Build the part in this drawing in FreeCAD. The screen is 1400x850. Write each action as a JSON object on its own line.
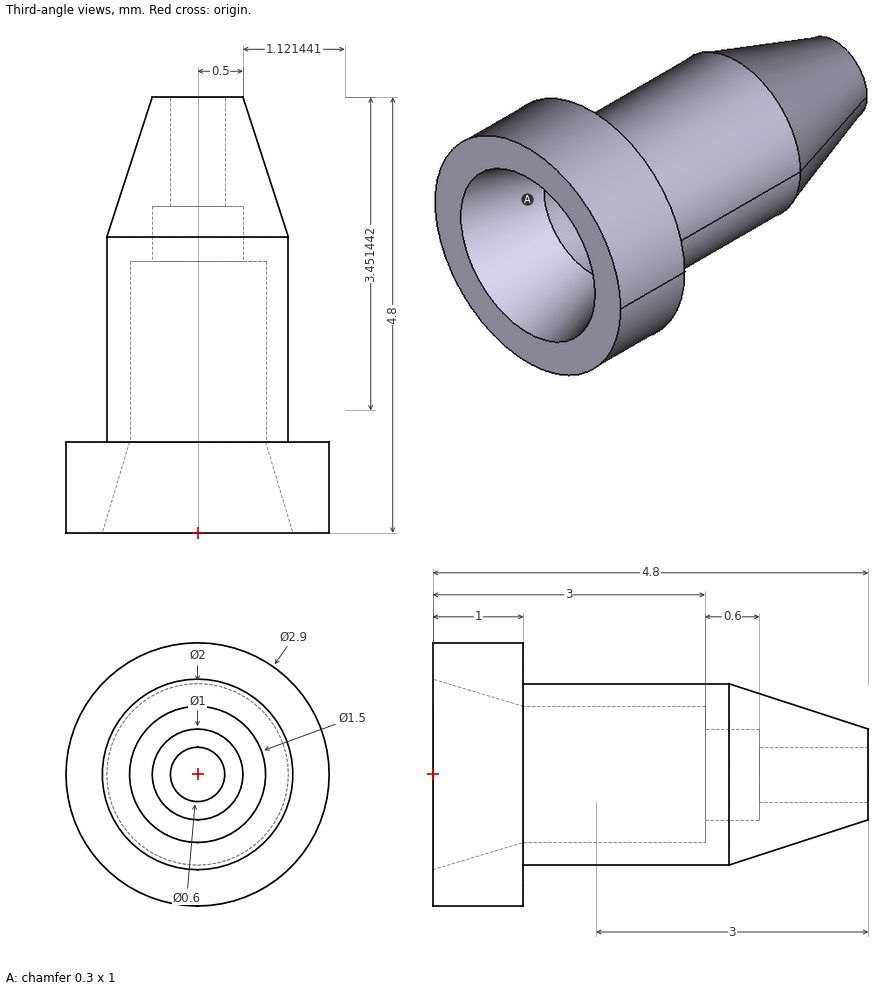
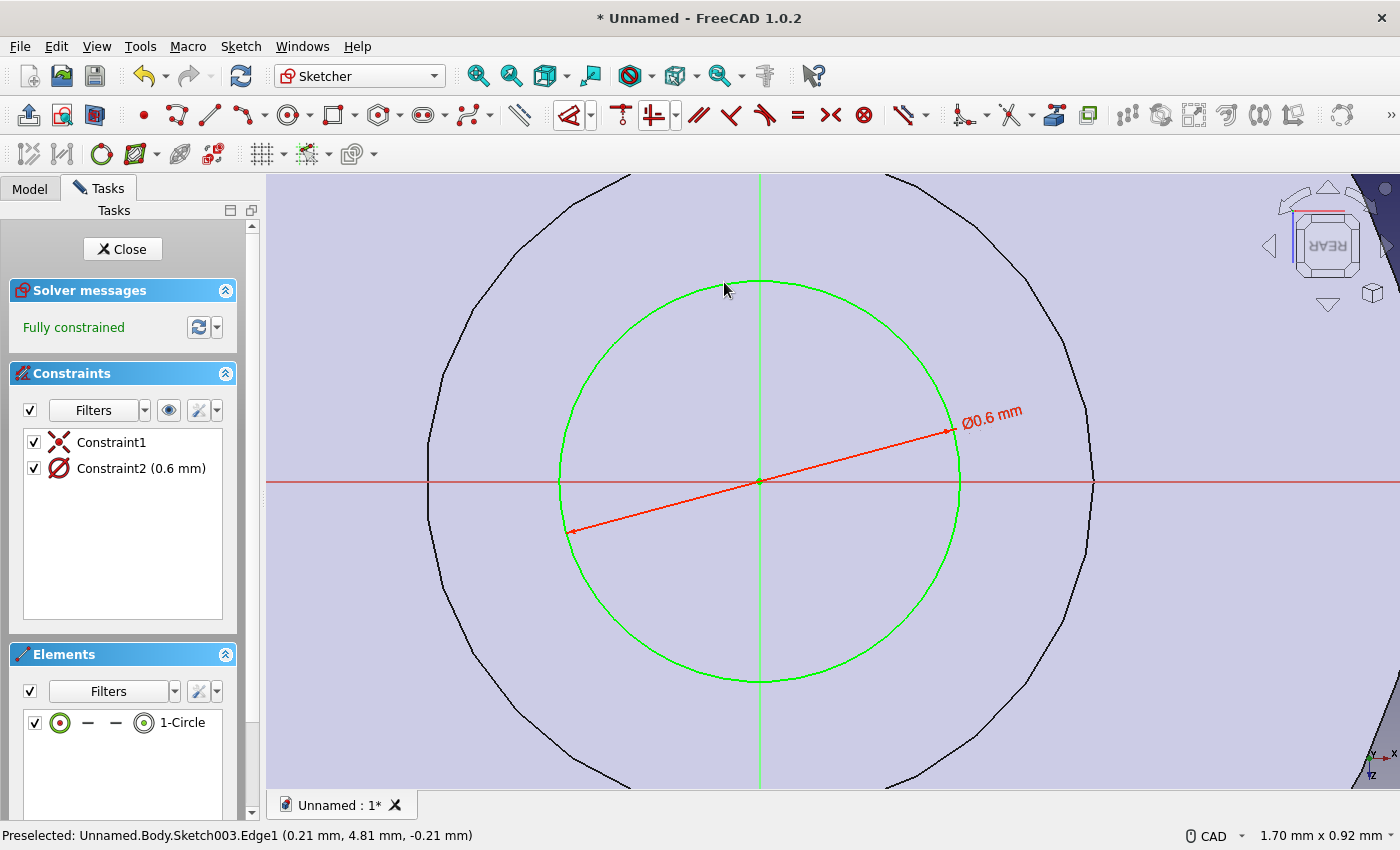
{"action": "left_click", "coordinate": [123, 249]}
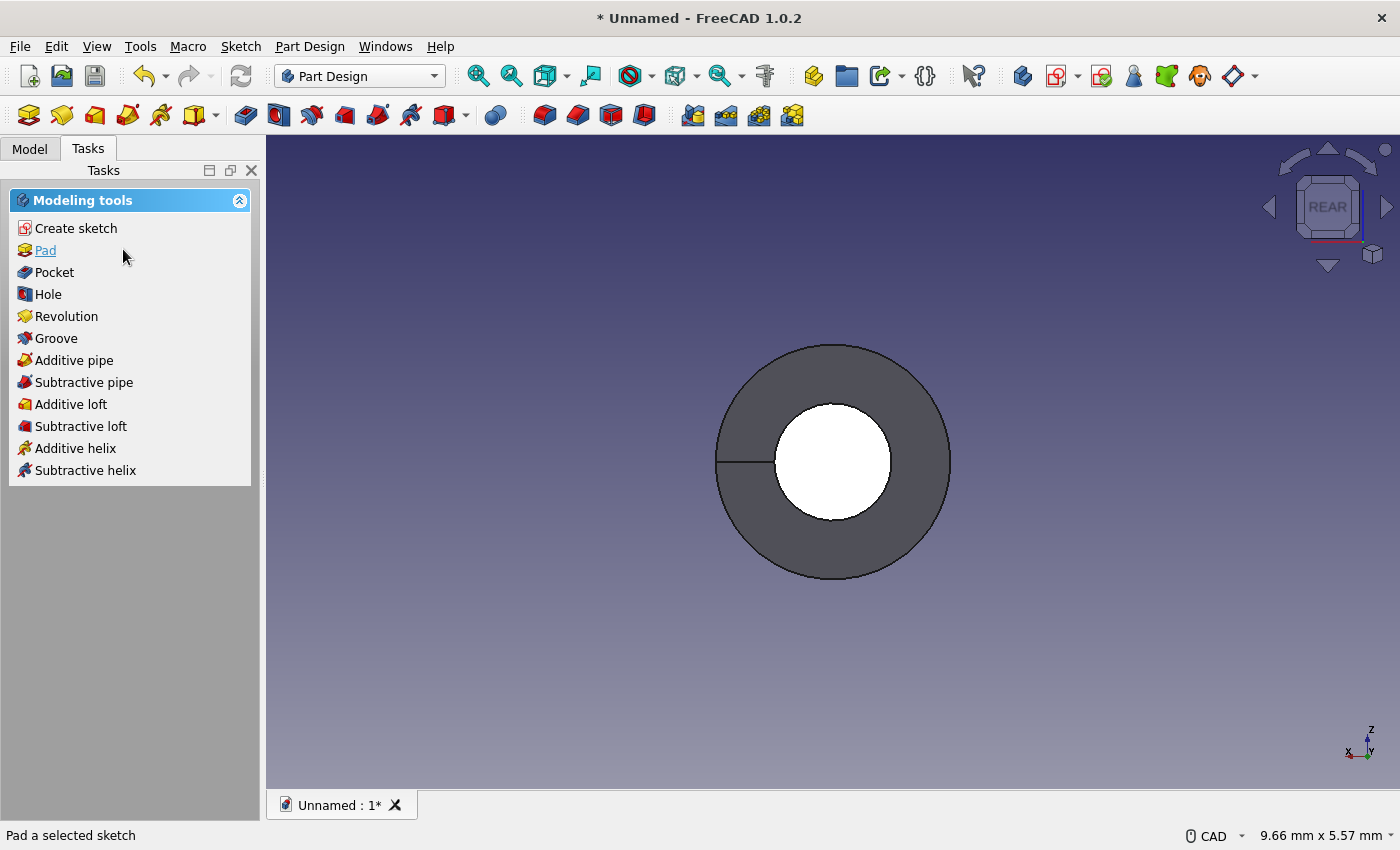
{"action": "left_click", "coordinate": [246, 116]}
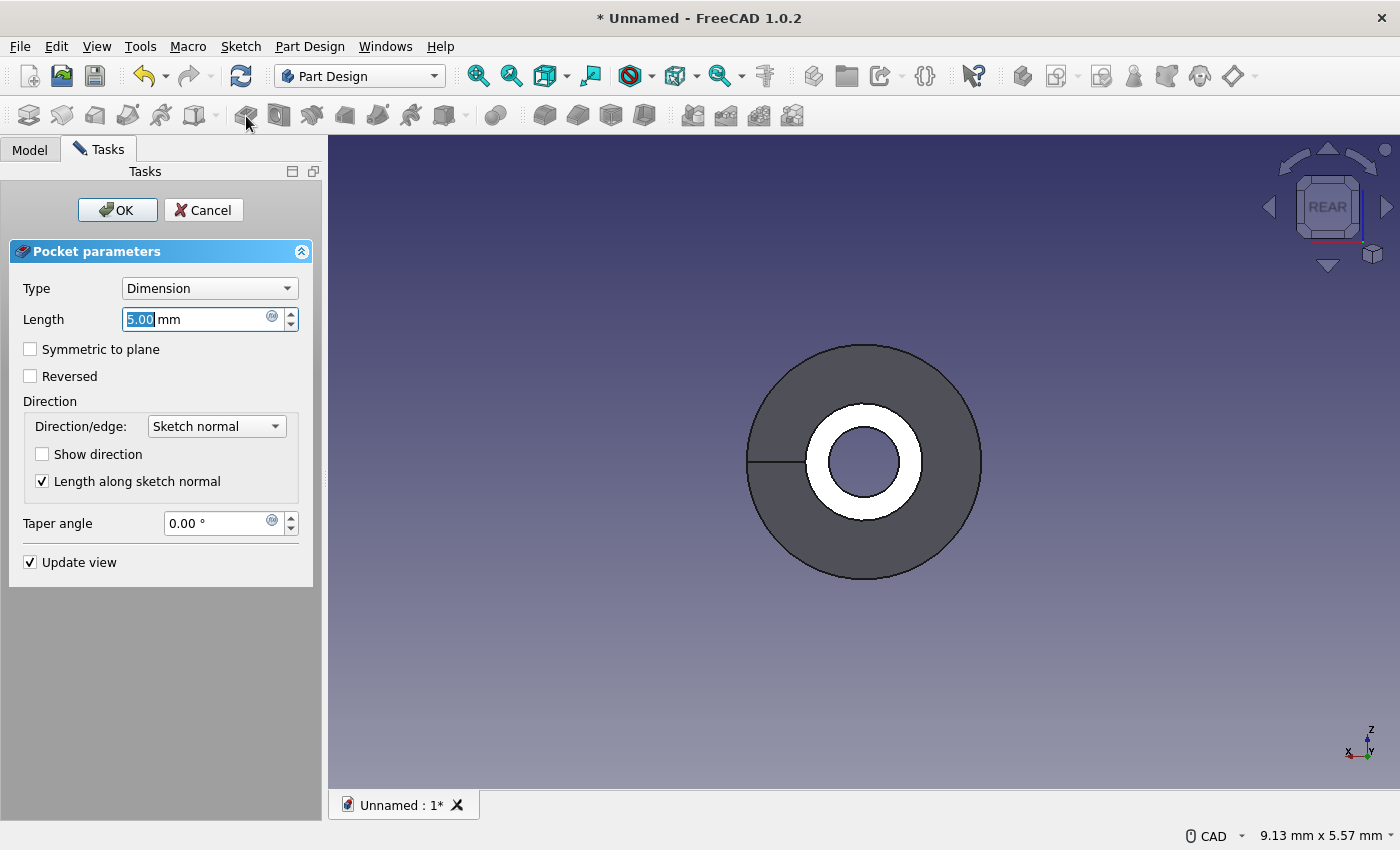
{"action": "type", "text": "3"}
{"action": "key", "text": "Tab"}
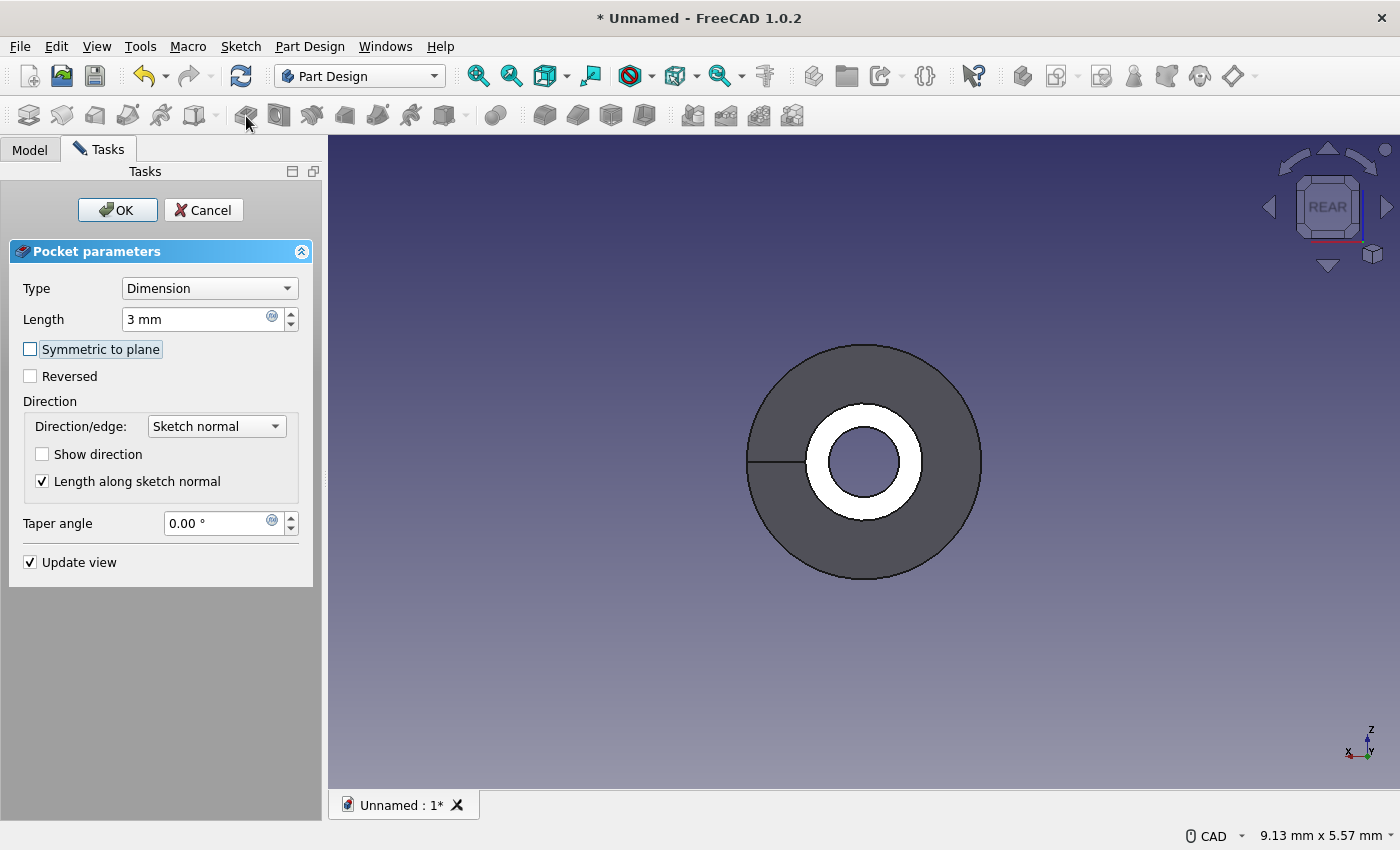
{"action": "left_click", "coordinate": [118, 210]}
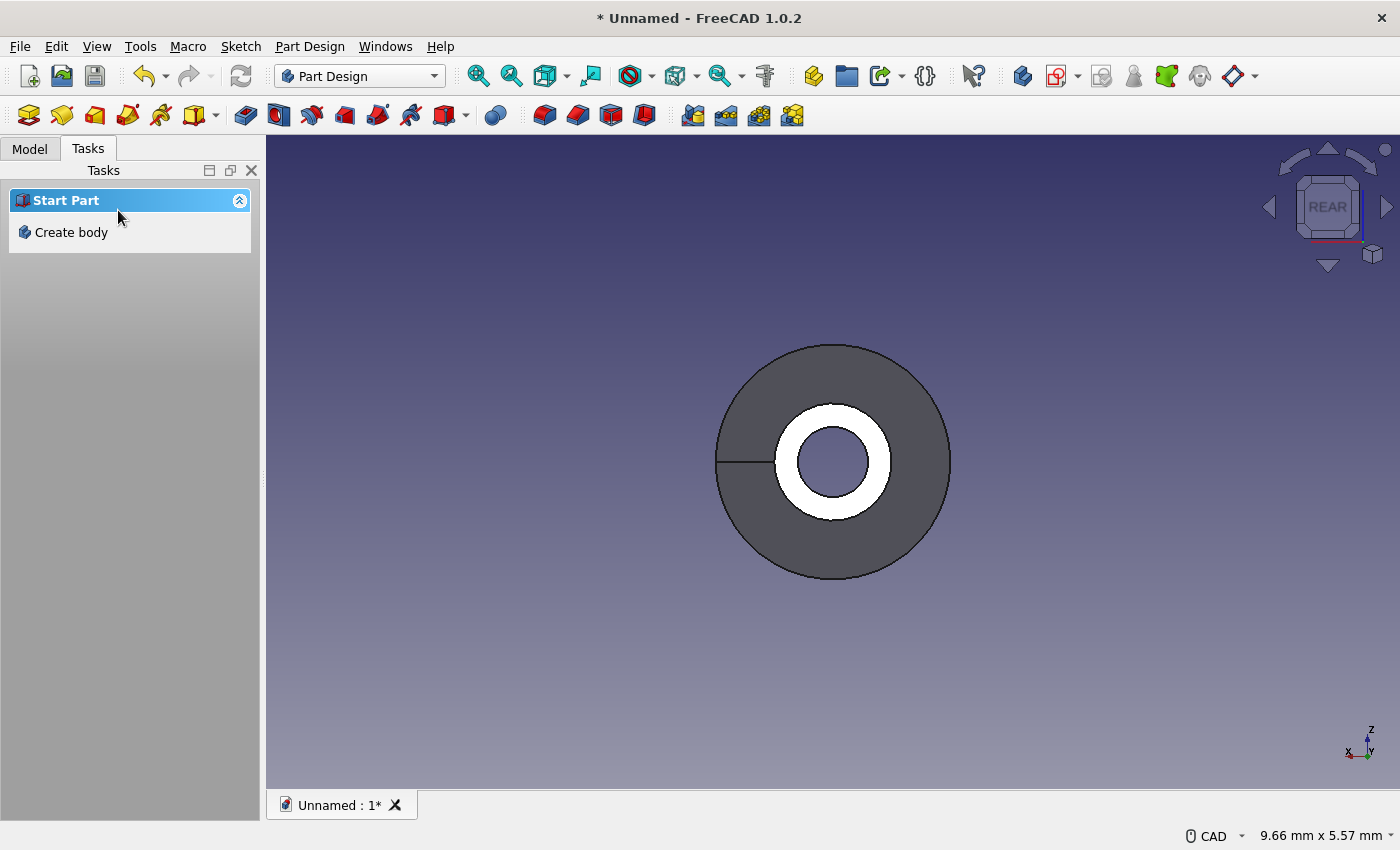
{"action": "key", "text": "v f"}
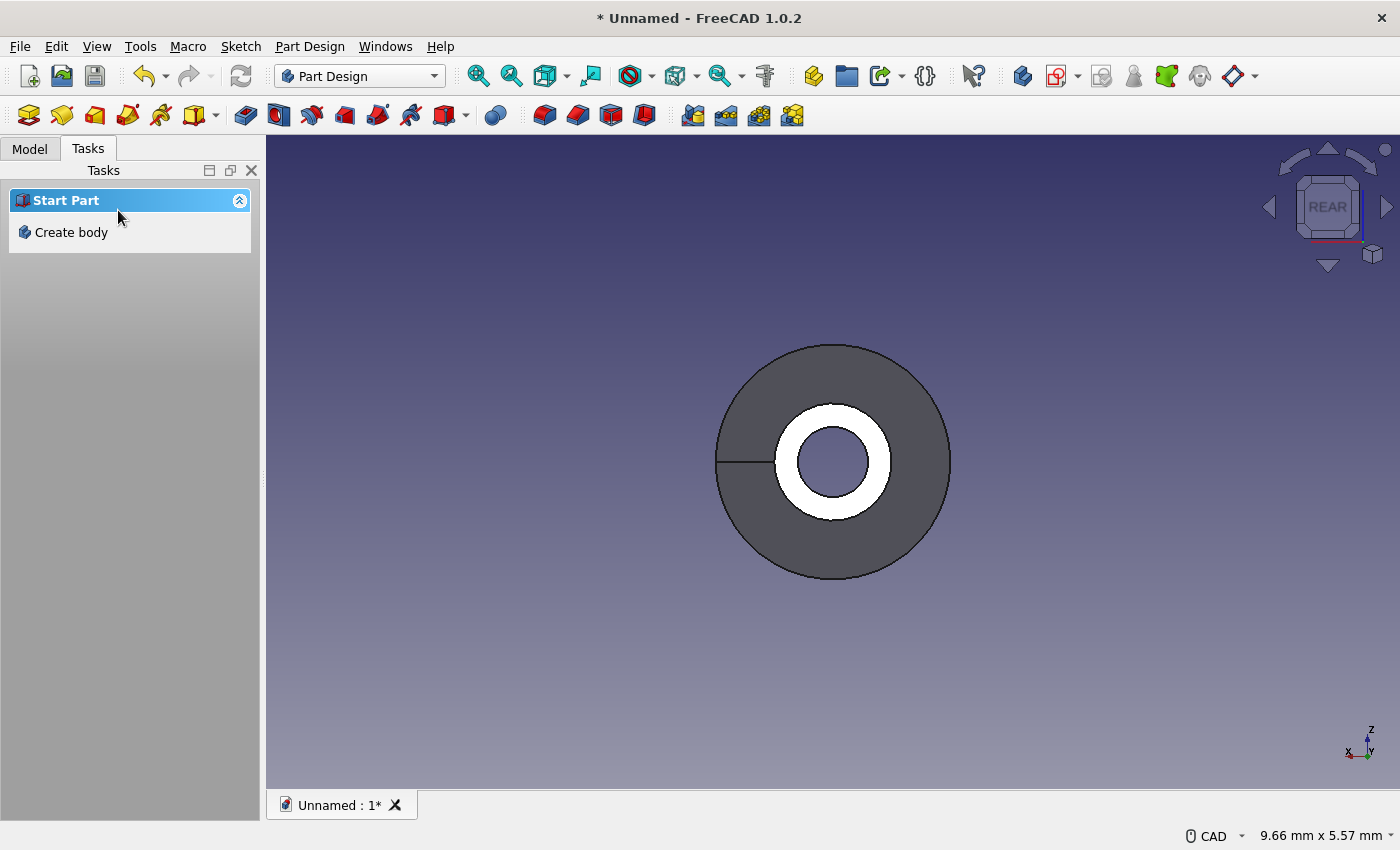
{"action": "key", "text": "0"}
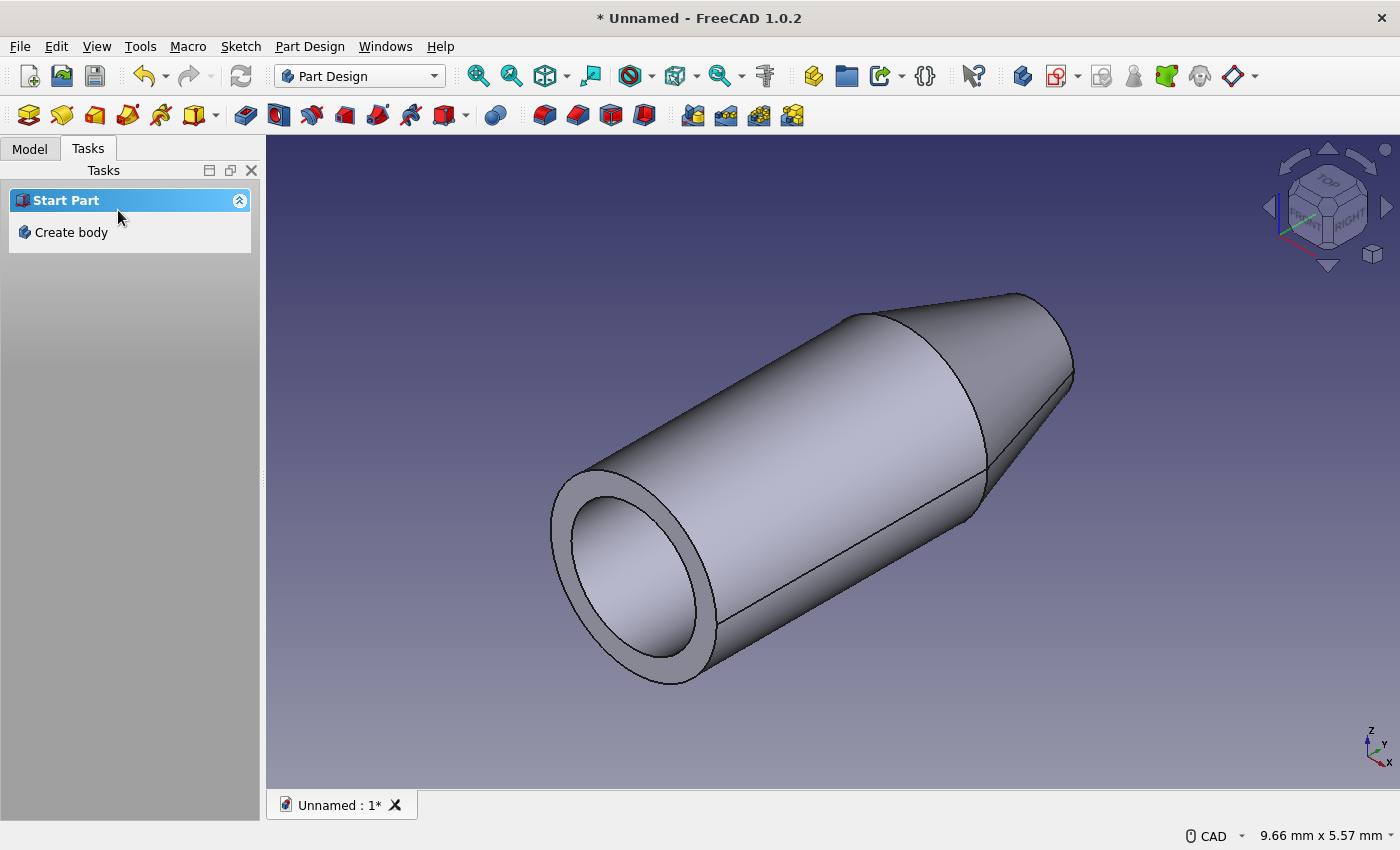
{"action": "key", "text": "1"}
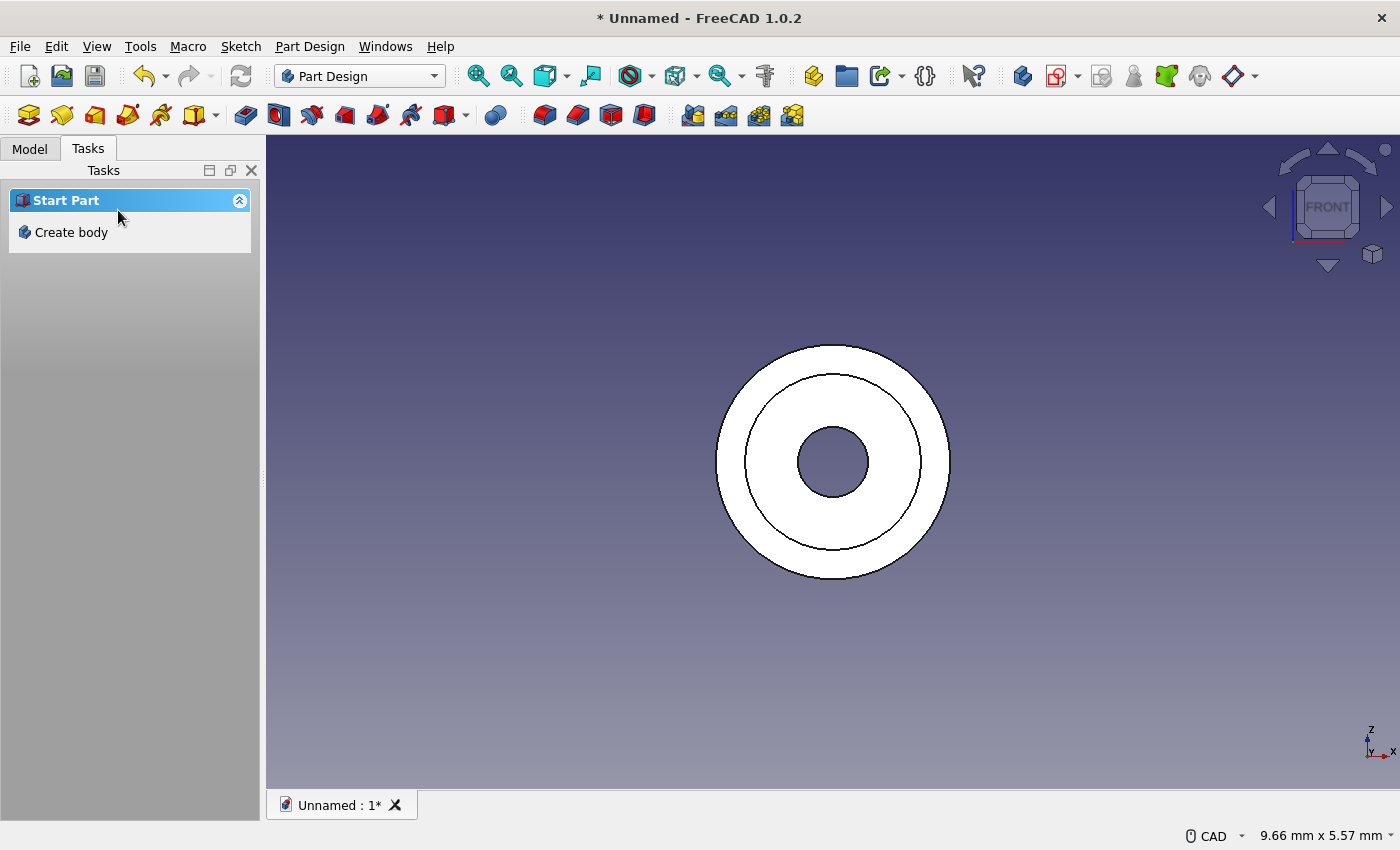
{"action": "left_click", "coordinate": [479, 76]}